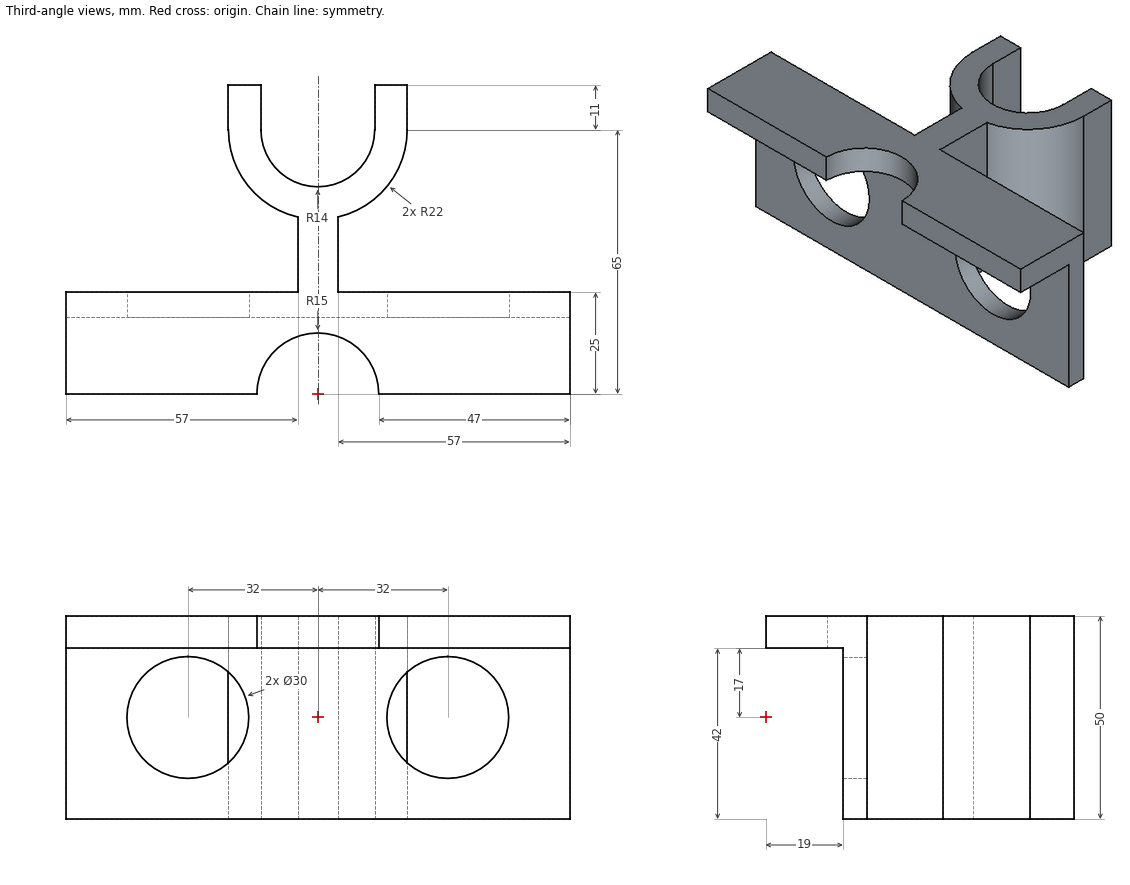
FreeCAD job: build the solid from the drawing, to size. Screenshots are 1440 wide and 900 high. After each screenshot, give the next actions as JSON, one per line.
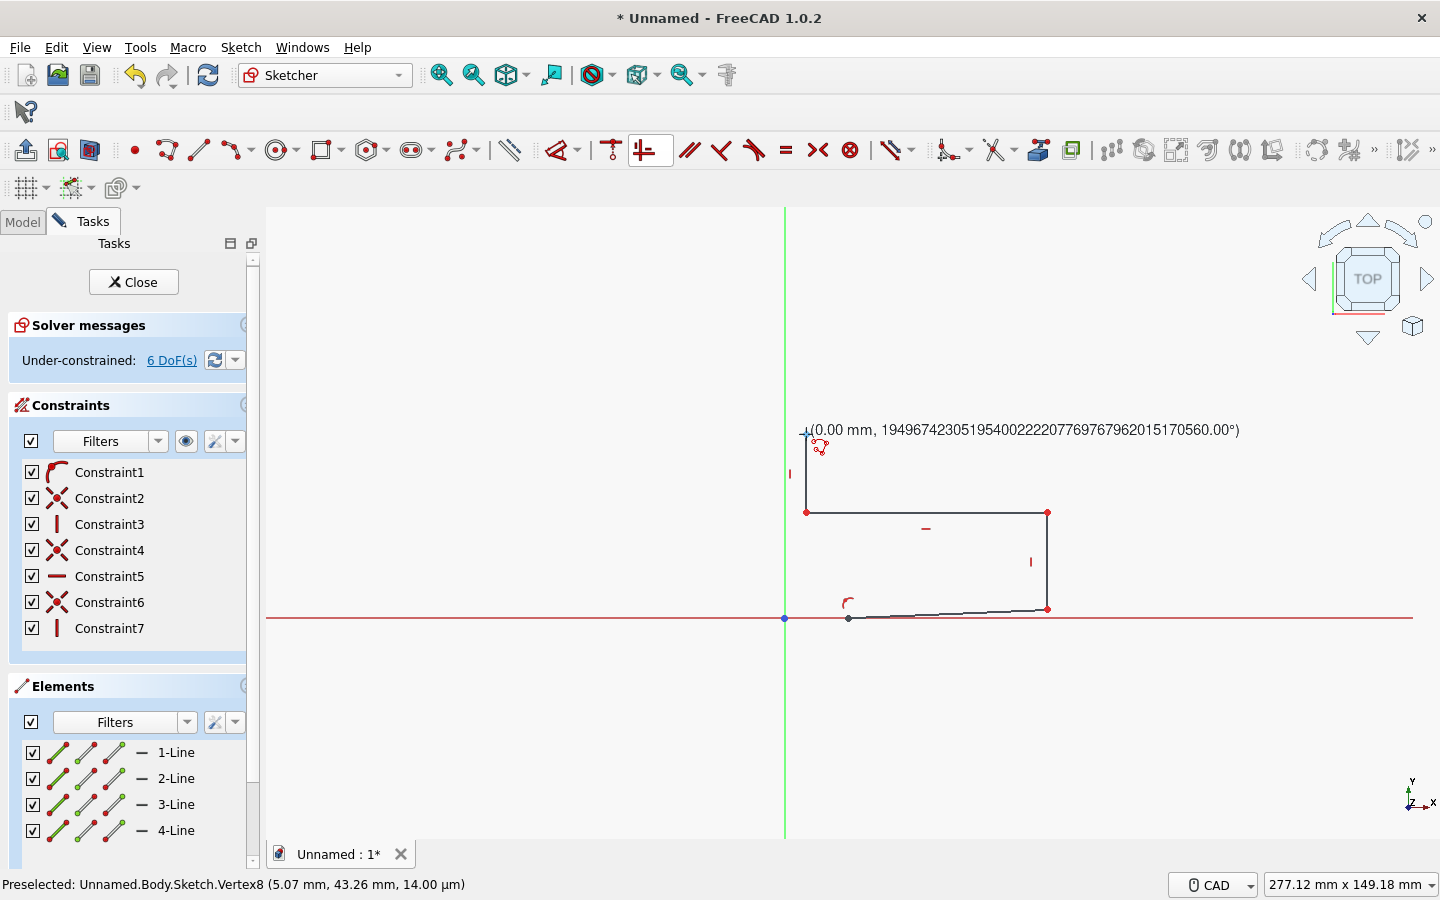
{"action": "left_click", "coordinate": [878, 343]}
{"action": "left_click", "coordinate": [878, 296]}
{"action": "left_click", "coordinate": [844, 296]}
{"action": "left_click", "coordinate": [844, 343]}
{"action": "right_click", "coordinate": [844, 343]}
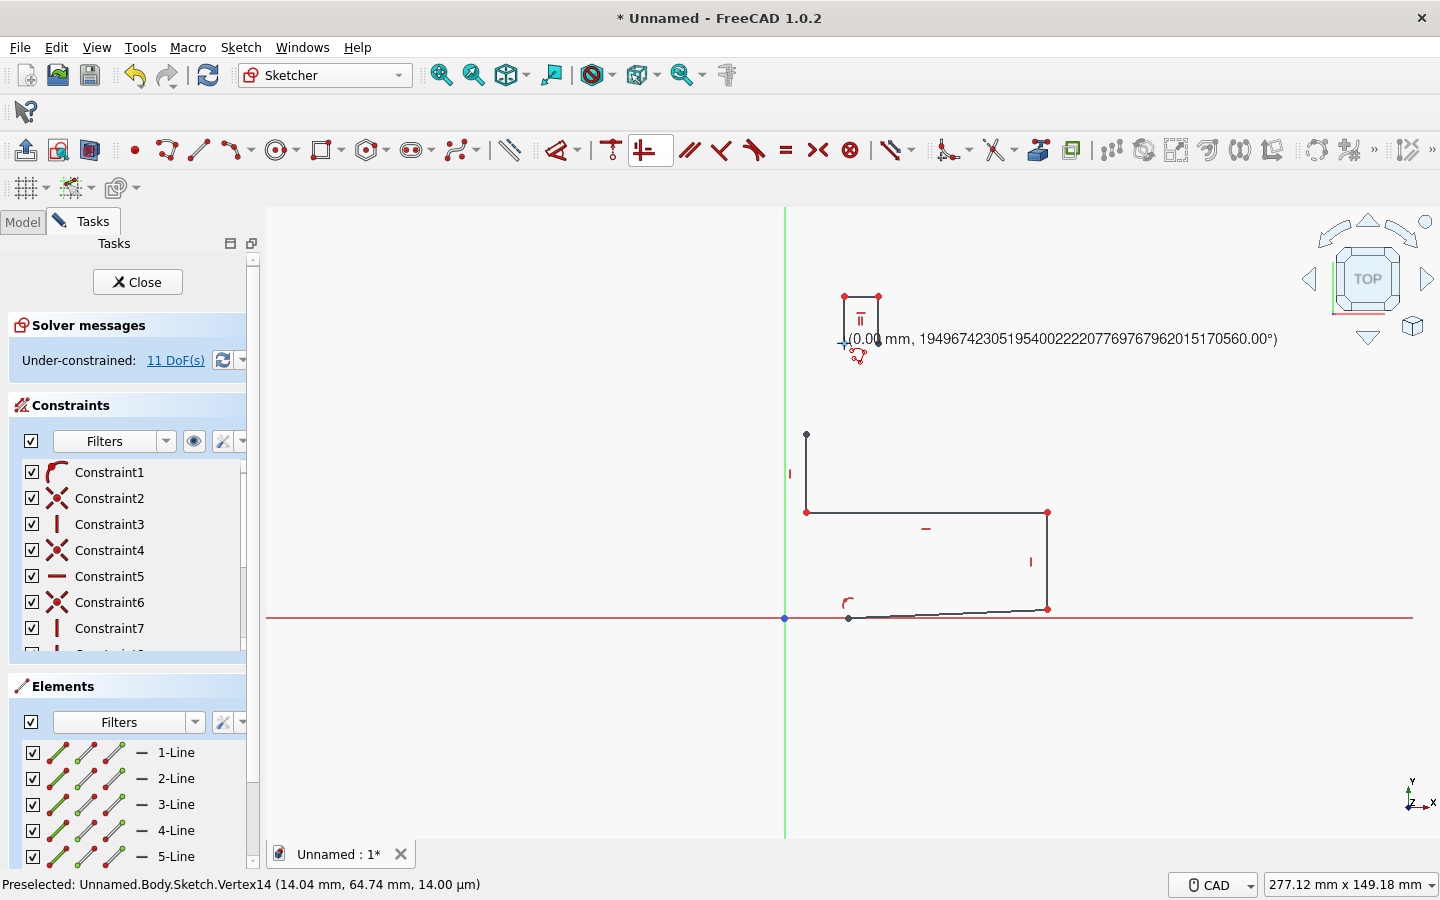
{"action": "left_click", "coordinate": [725, 343]}
{"action": "left_click", "coordinate": [725, 296]}
{"action": "left_click", "coordinate": [691, 296]}
{"action": "left_click", "coordinate": [691, 343]}
{"action": "right_click", "coordinate": [691, 343]}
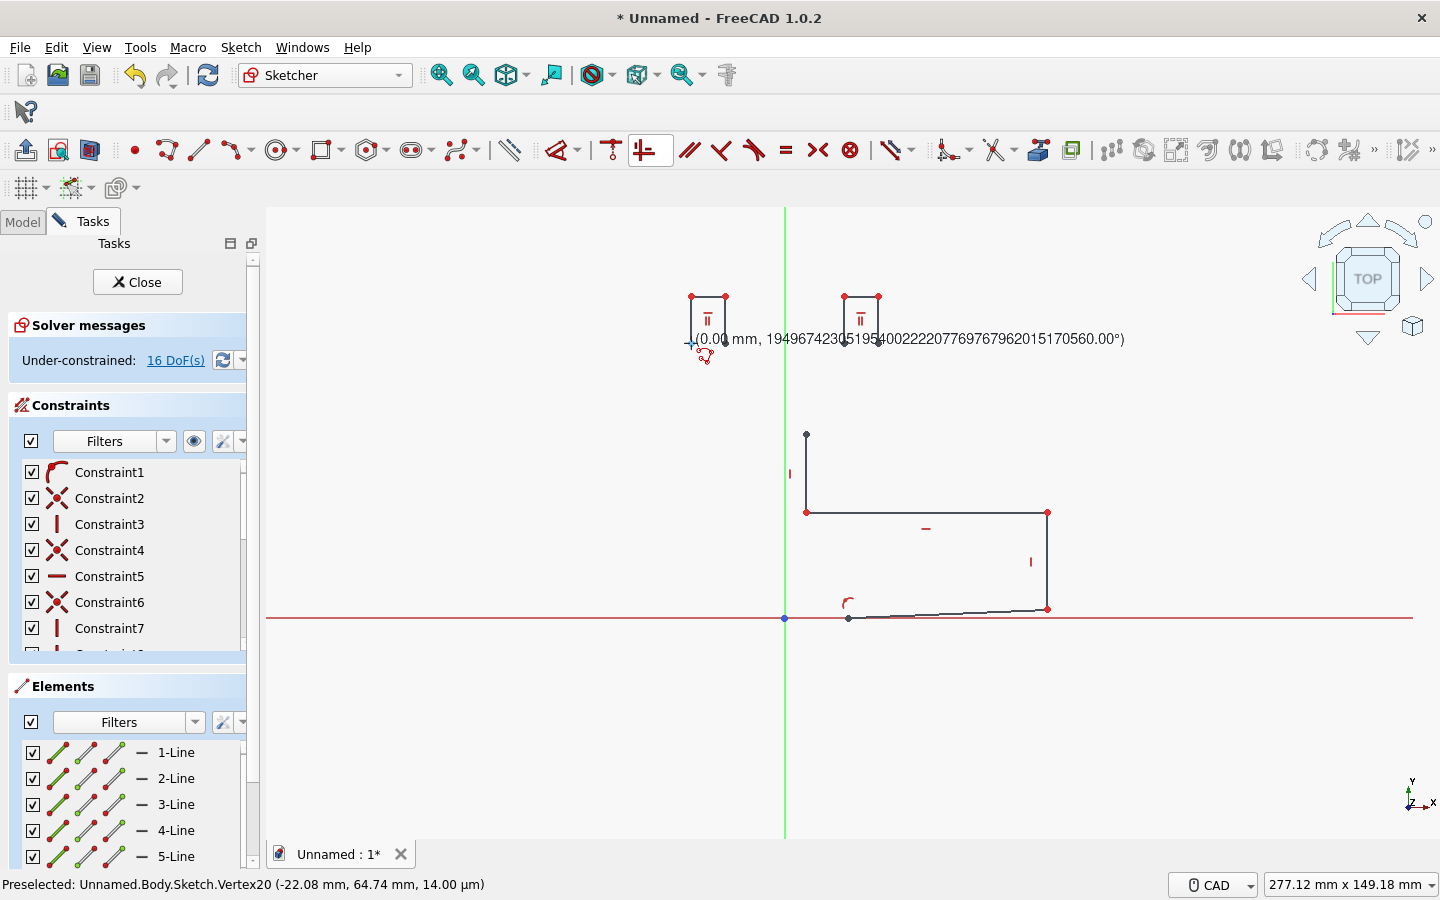
{"action": "left_click", "coordinate": [763, 434]}
{"action": "left_click", "coordinate": [763, 512]}
{"action": "left_click", "coordinate": [522, 512]}
{"action": "left_click", "coordinate": [522, 618]}
{"action": "left_click", "coordinate": [721, 609]}
{"action": "right_click", "coordinate": [721, 609]}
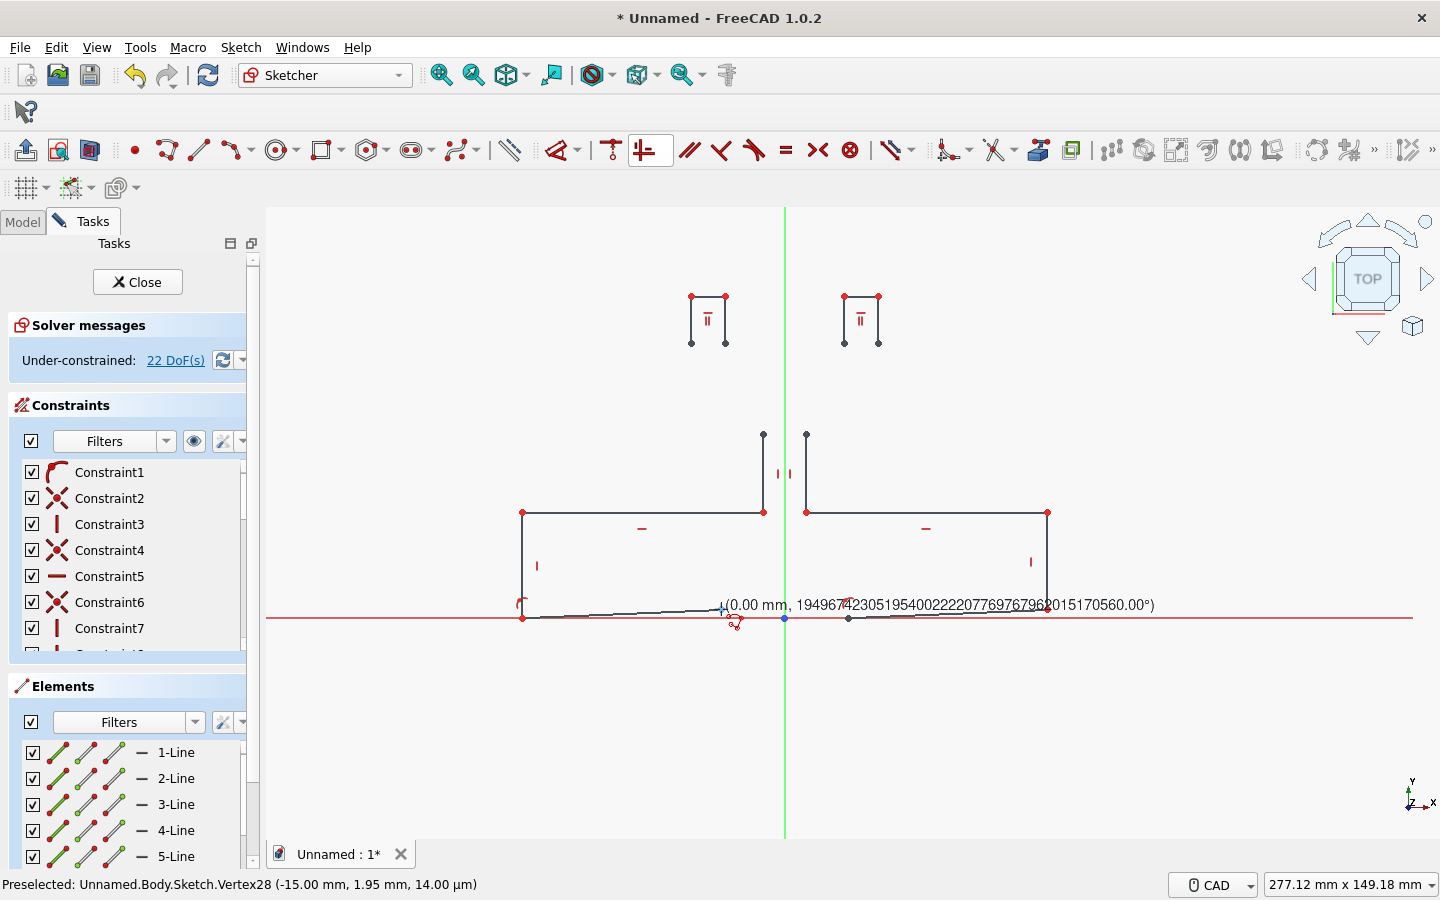
{"action": "left_click", "coordinate": [232, 150]}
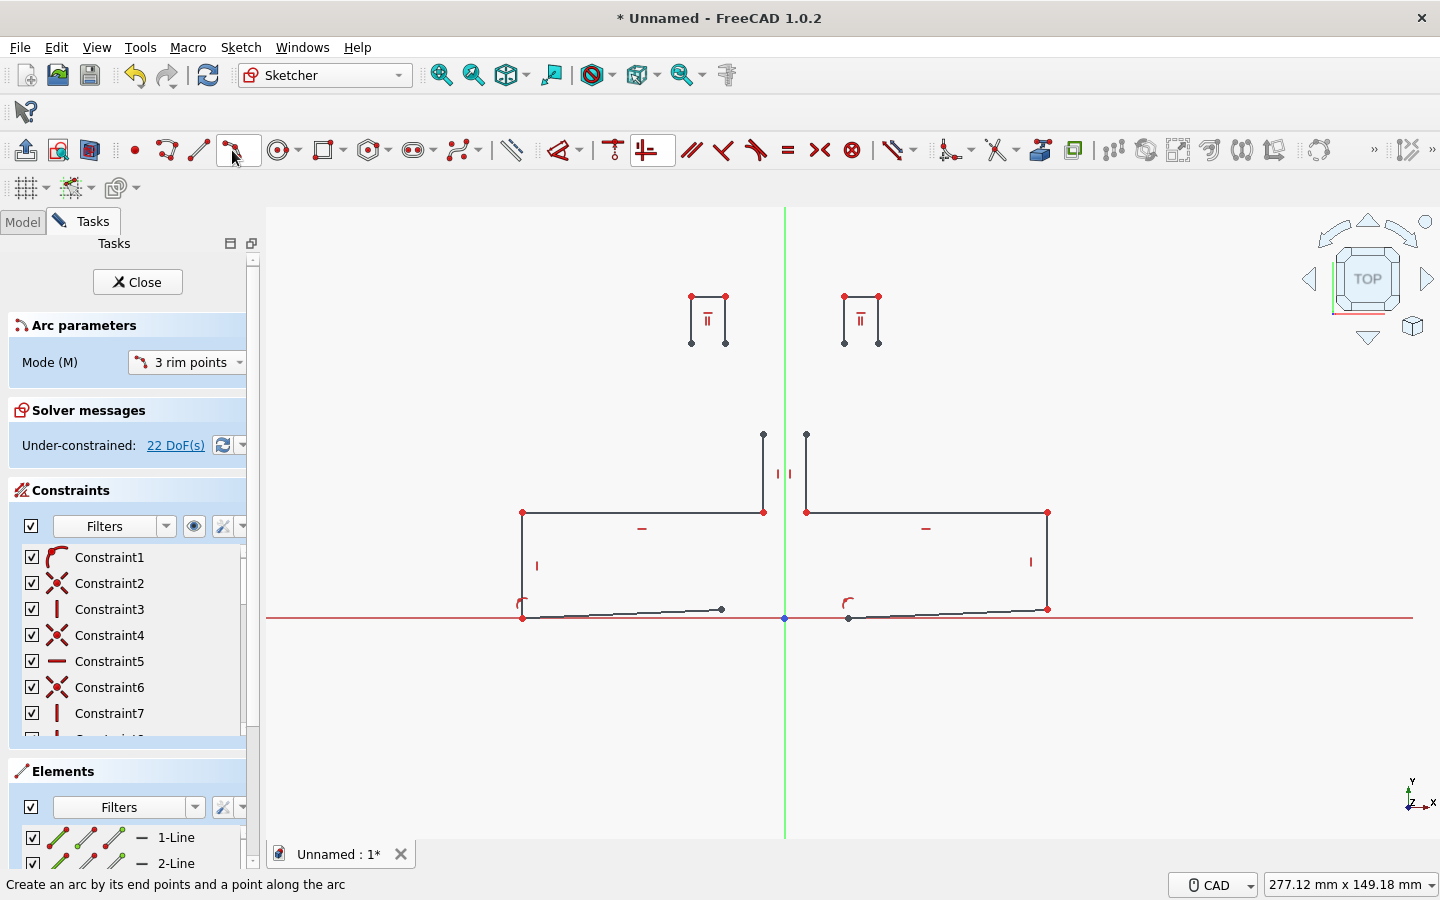
{"action": "left_click", "coordinate": [806, 435]}
{"action": "left_click", "coordinate": [878, 344]}
{"action": "left_click", "coordinate": [858, 401]}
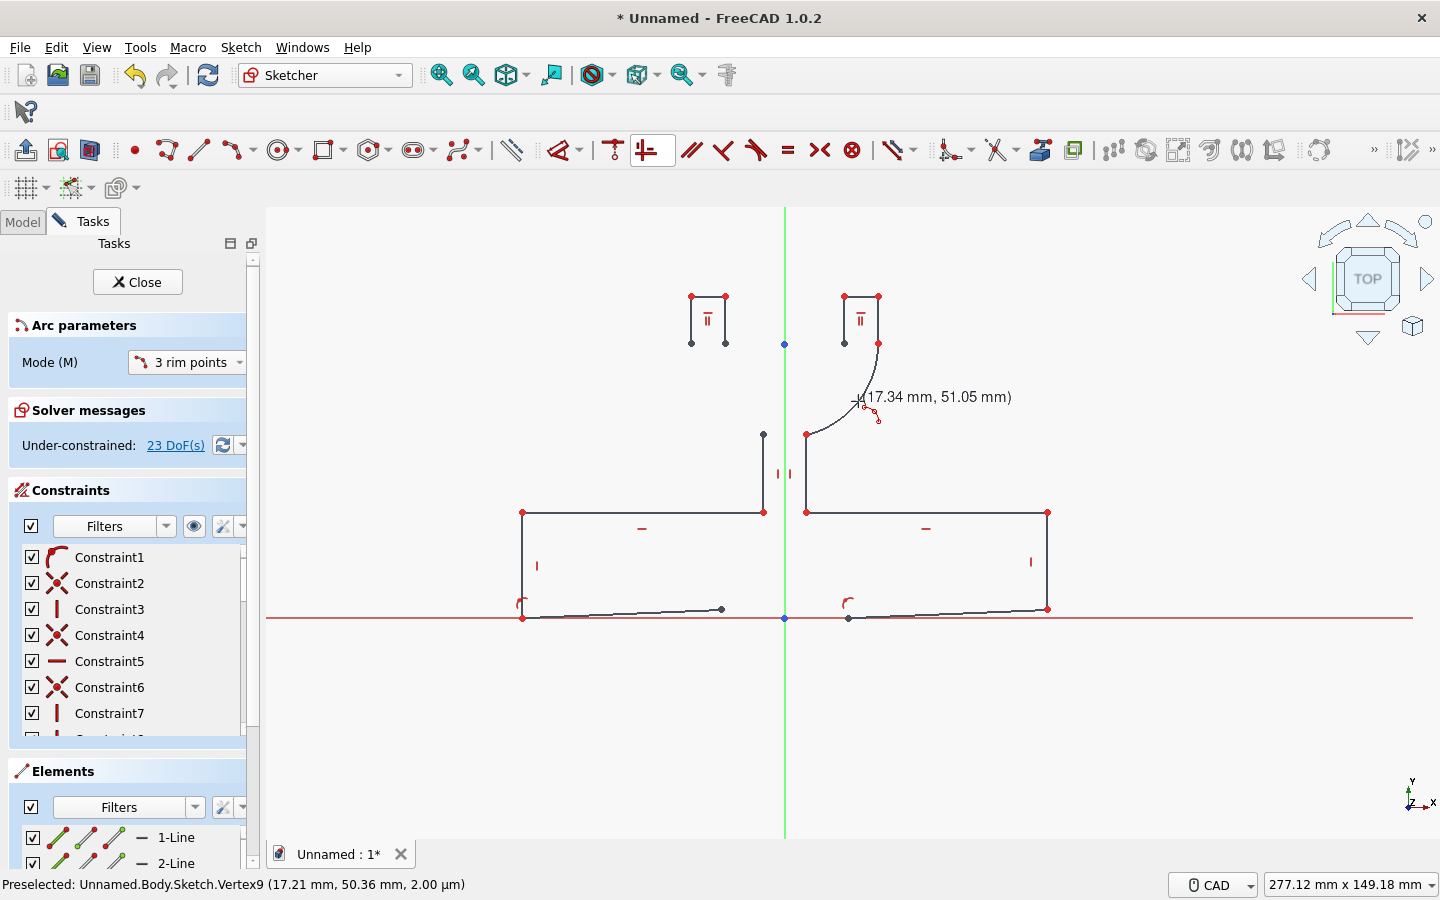
{"action": "left_click", "coordinate": [844, 344]}
{"action": "left_click", "coordinate": [725, 344]}
{"action": "left_click", "coordinate": [766, 399]}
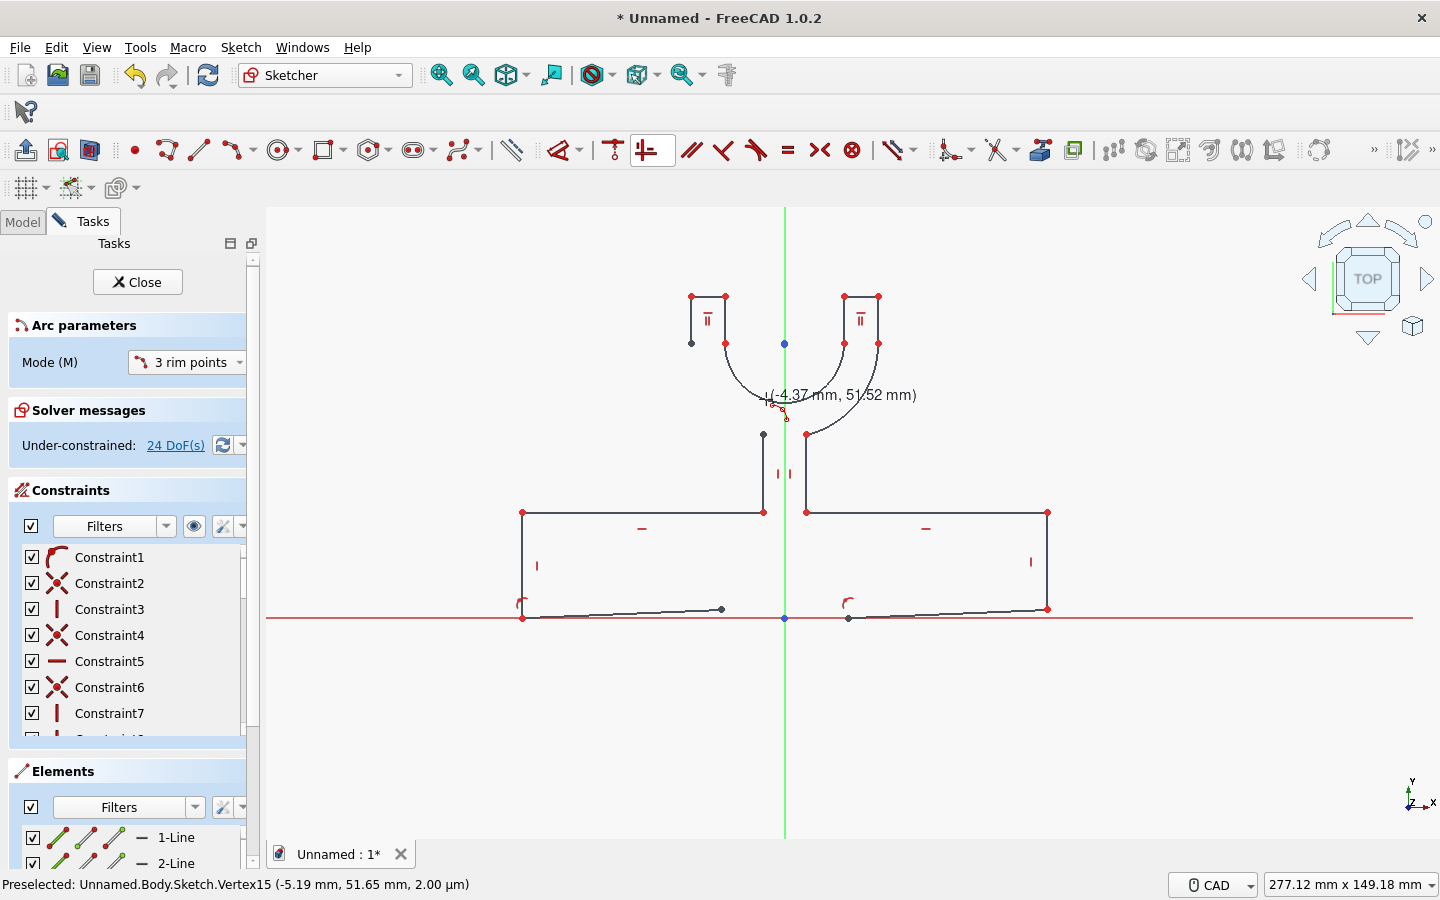
{"action": "left_click", "coordinate": [691, 344]}
{"action": "left_click", "coordinate": [763, 435]}
{"action": "left_click", "coordinate": [712, 401]}